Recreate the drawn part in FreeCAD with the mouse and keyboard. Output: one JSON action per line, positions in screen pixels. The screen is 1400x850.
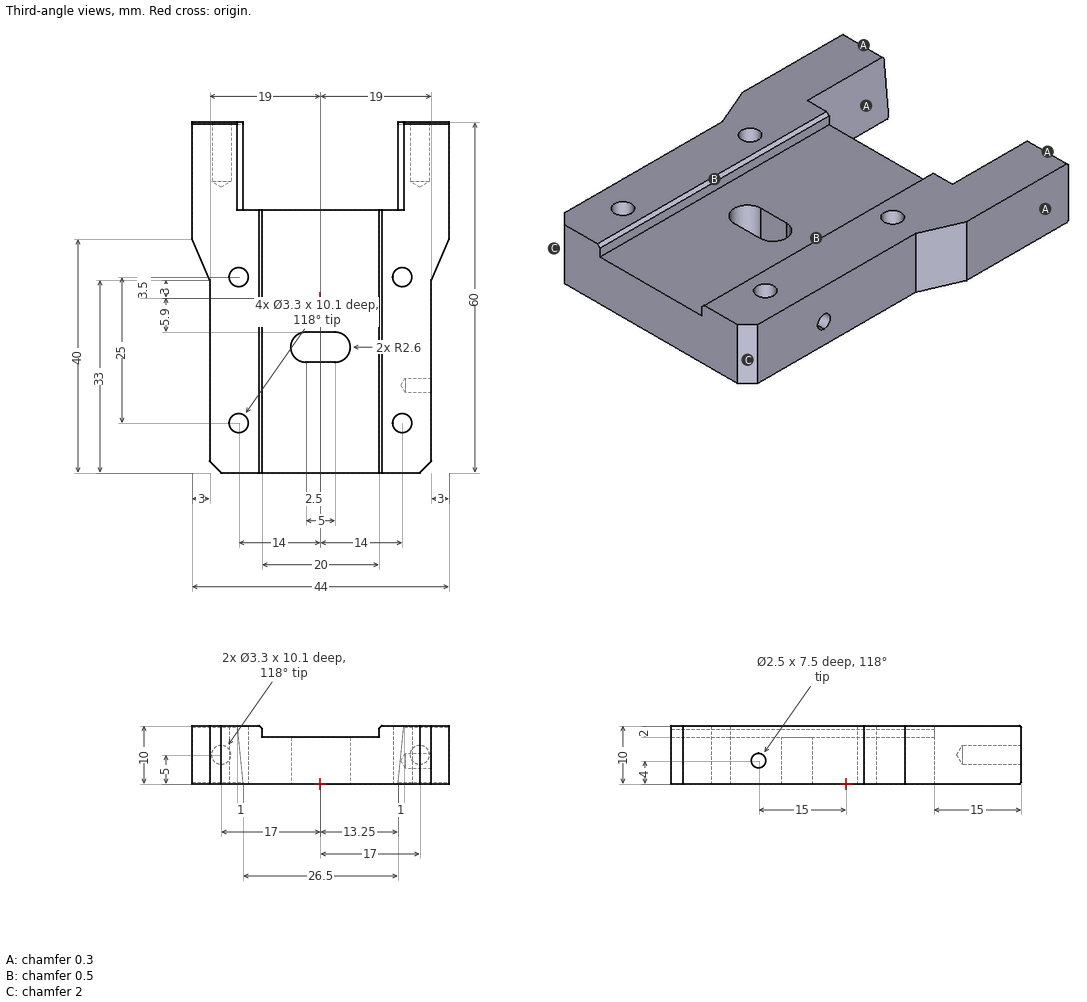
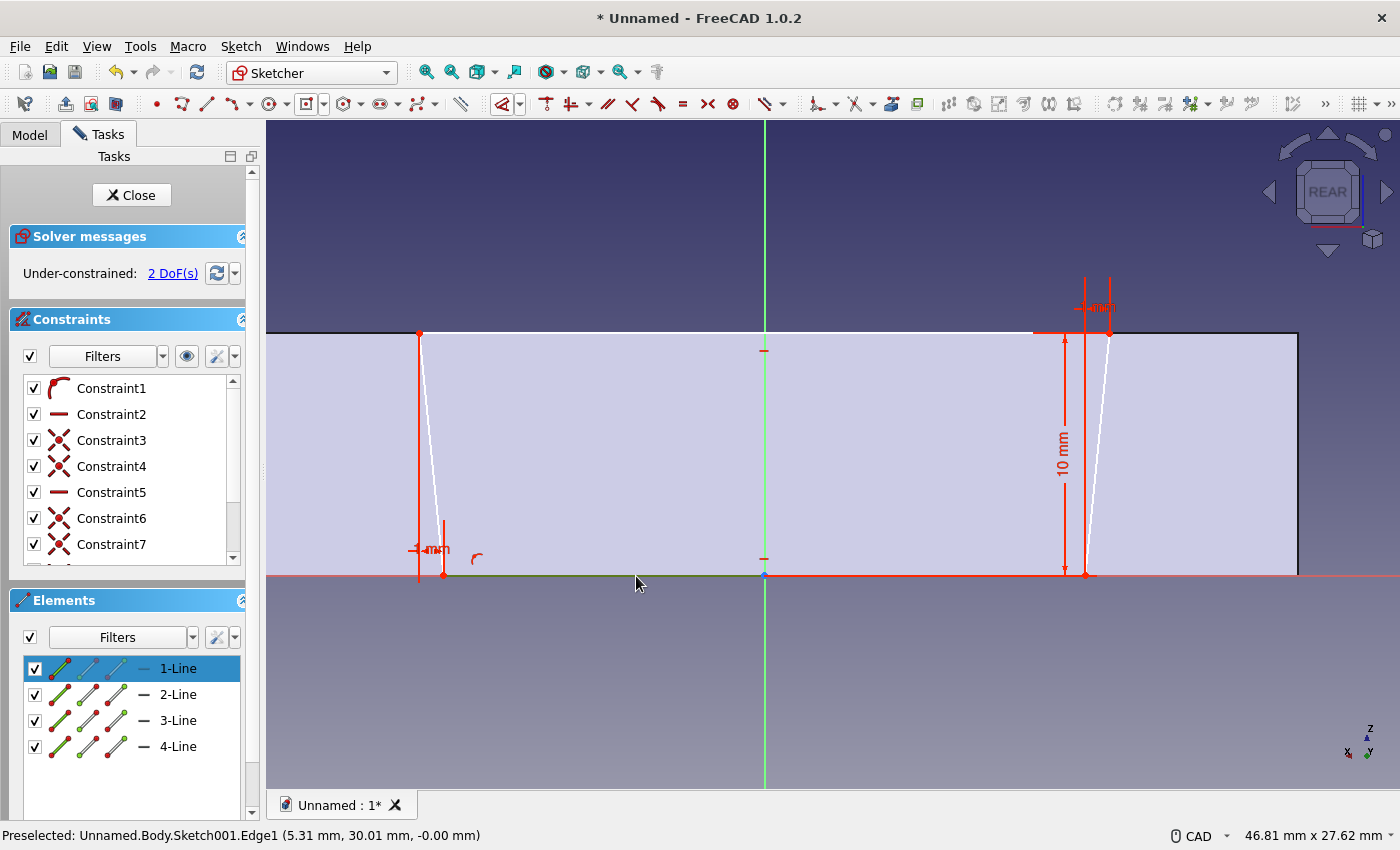
{"action": "left_click", "coordinate": [520, 104]}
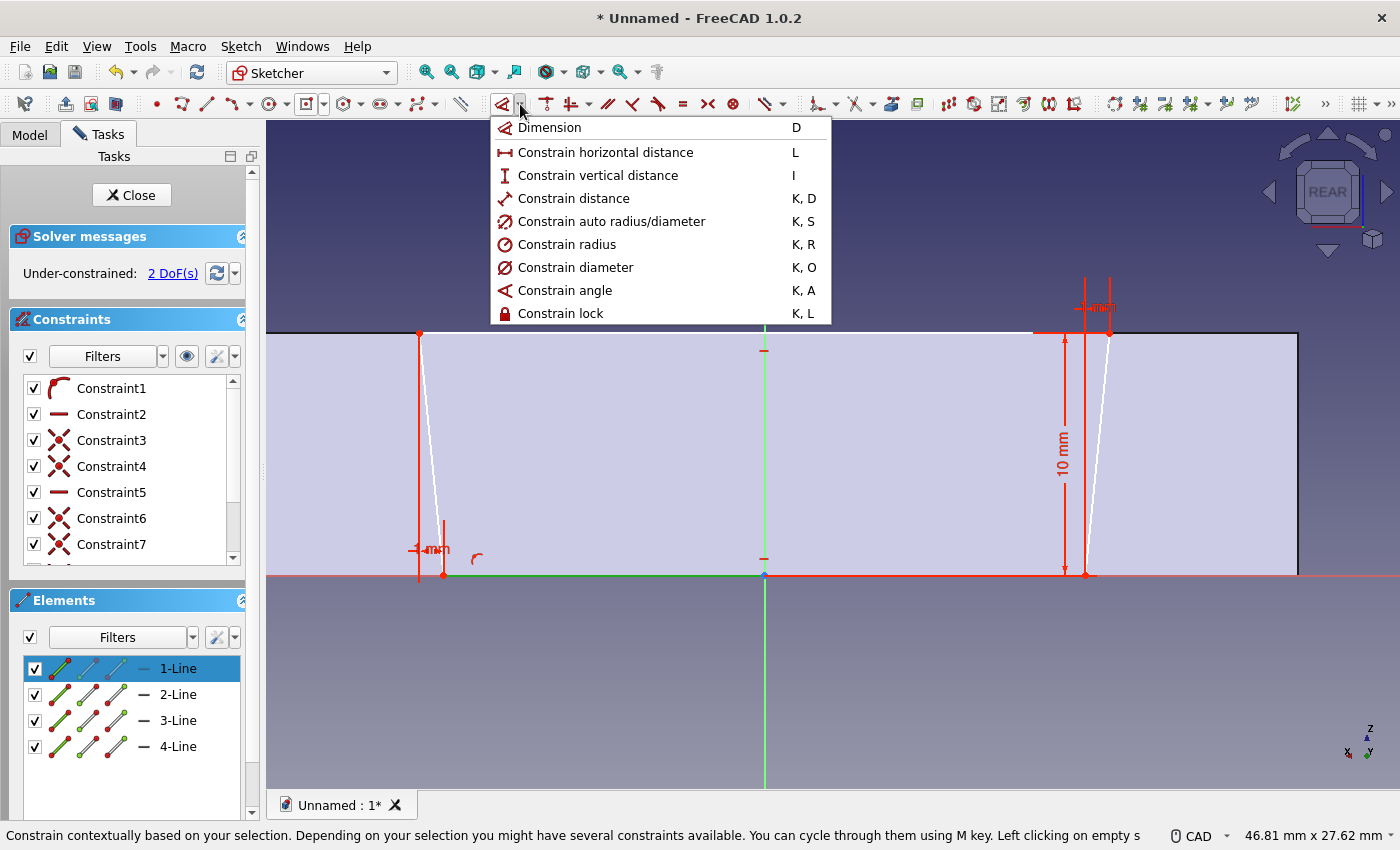
{"action": "left_click", "coordinate": [661, 152]}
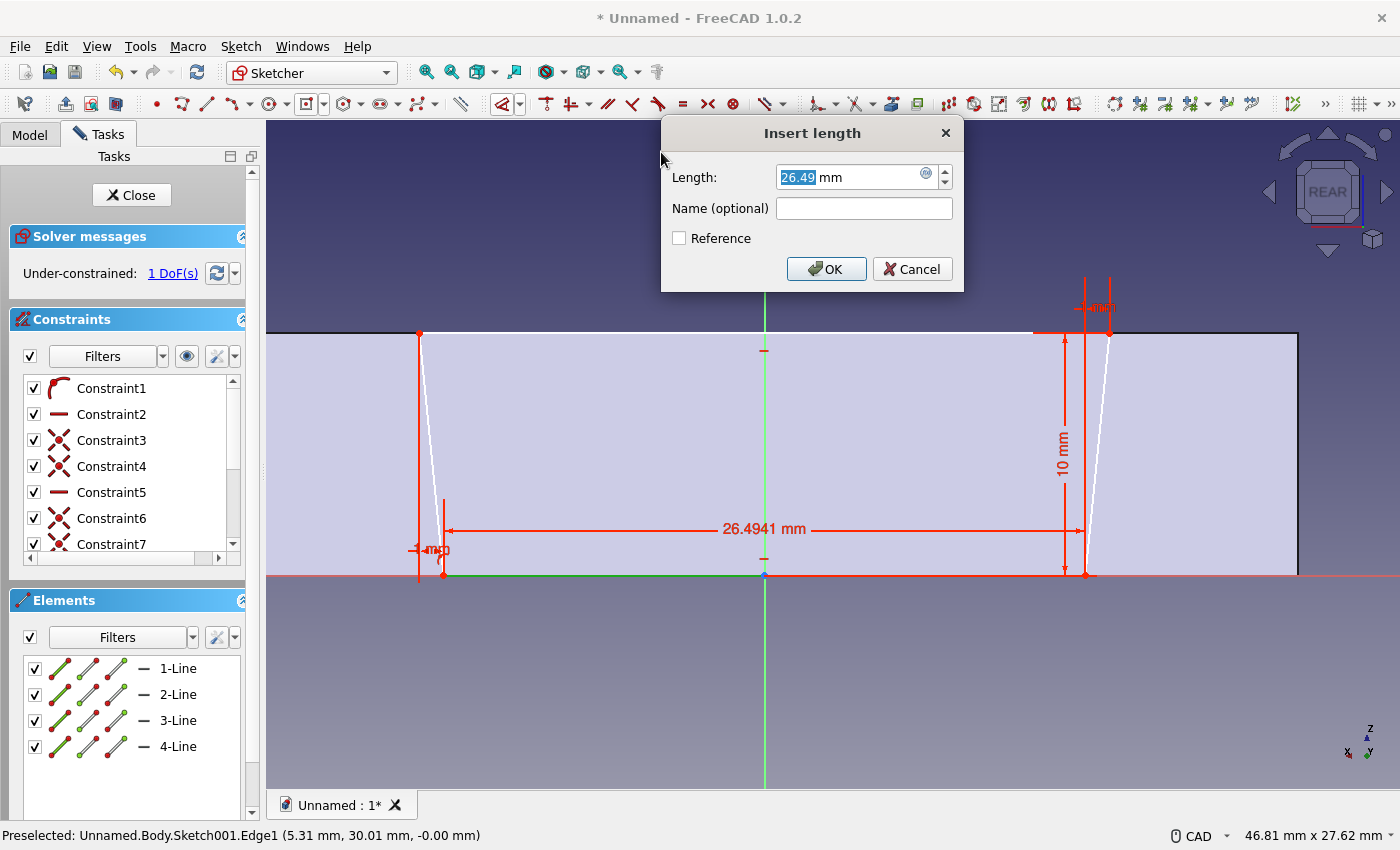
{"action": "type", "text": "26.5"}
{"action": "key", "text": "Return"}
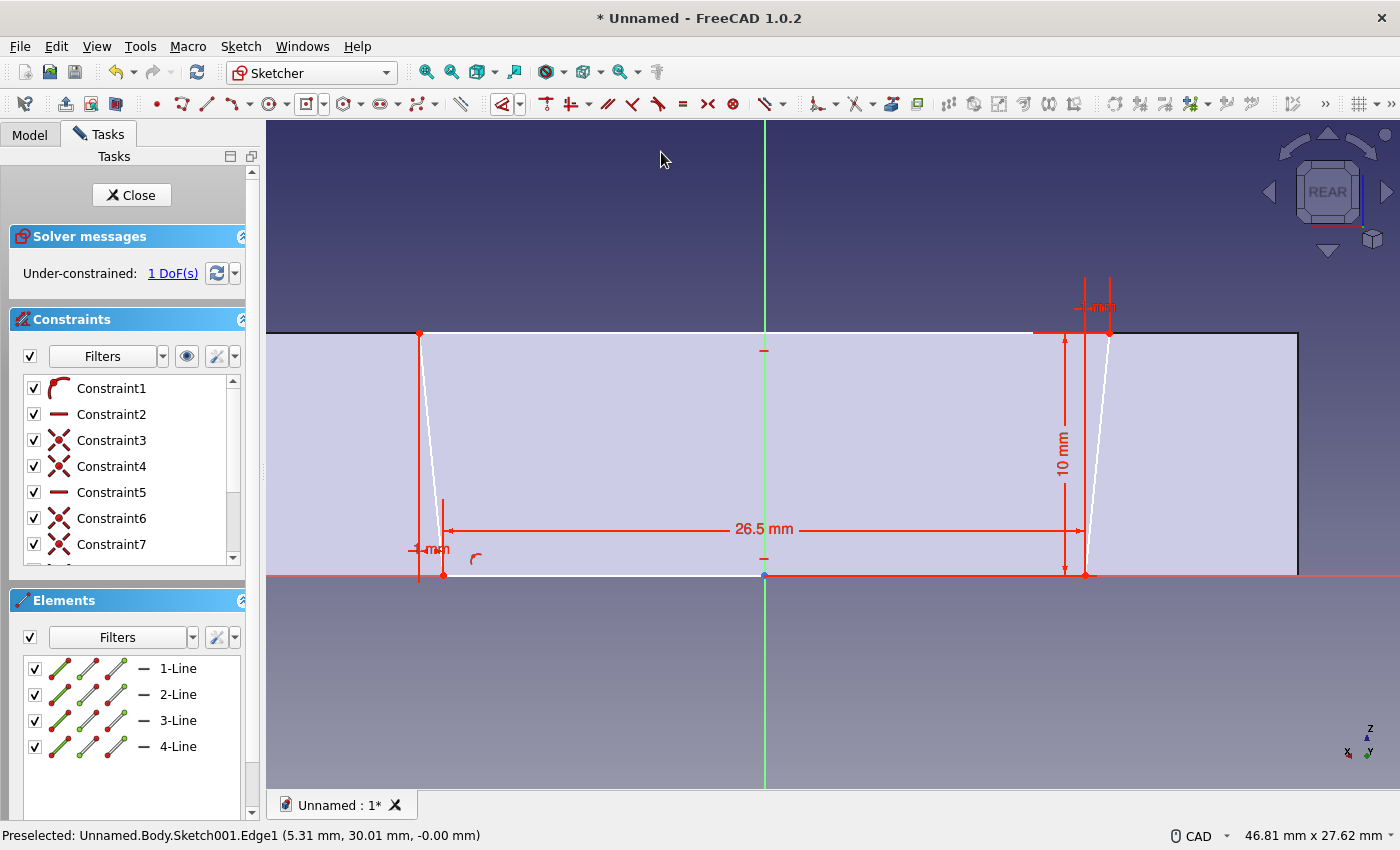
{"action": "left_click", "coordinate": [443, 576]}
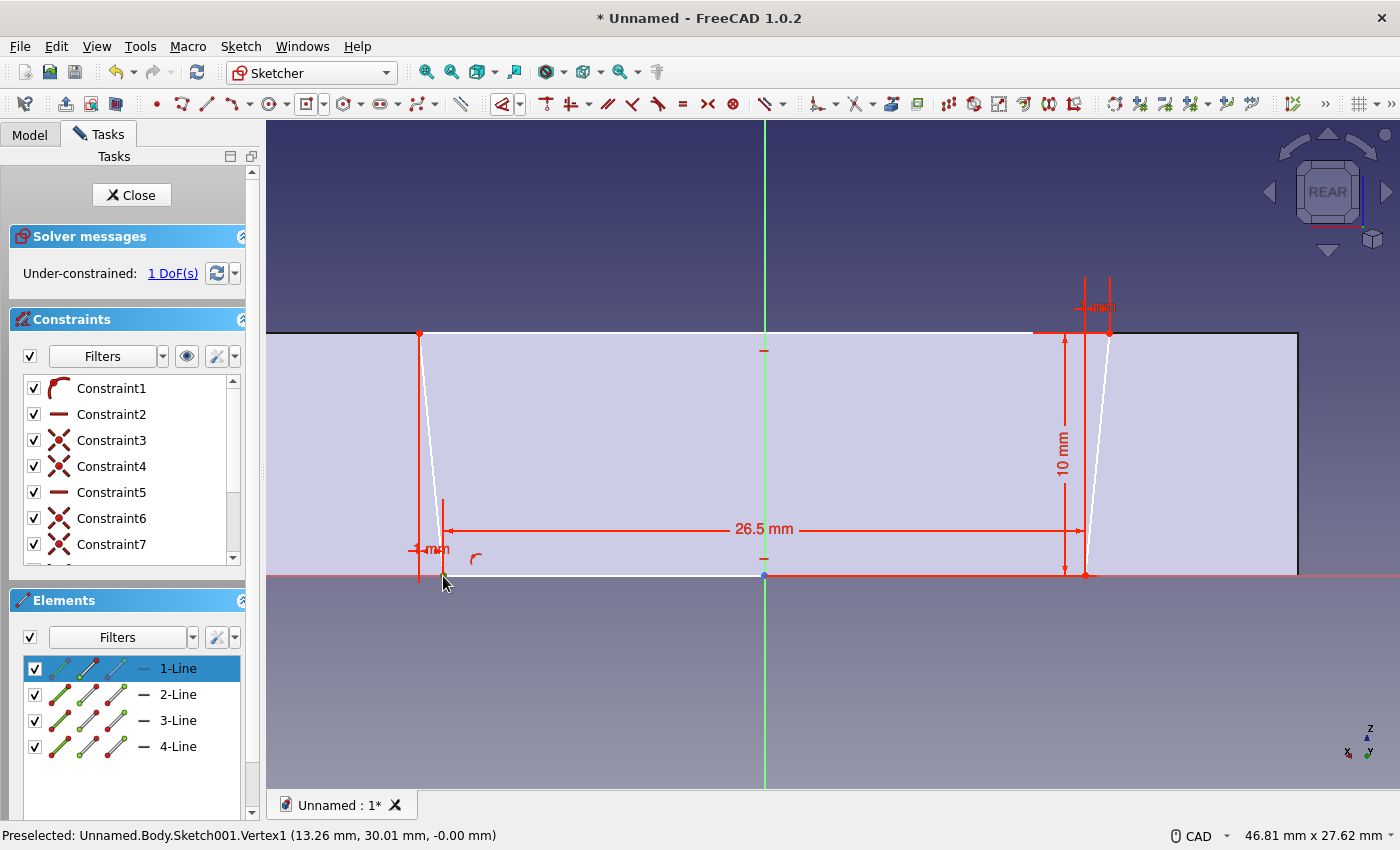
{"action": "left_click", "coordinate": [520, 104]}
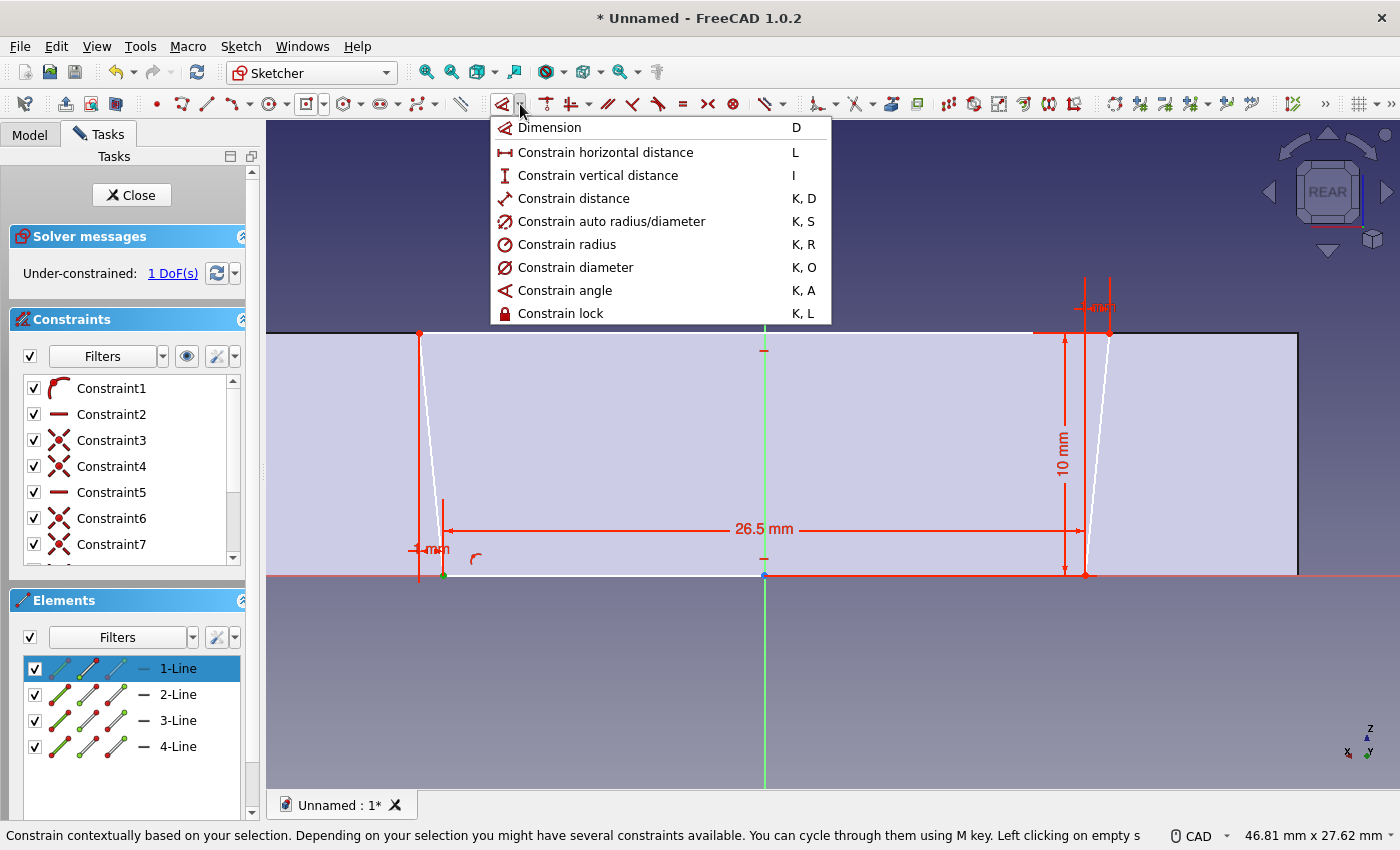
{"action": "left_click", "coordinate": [661, 152]}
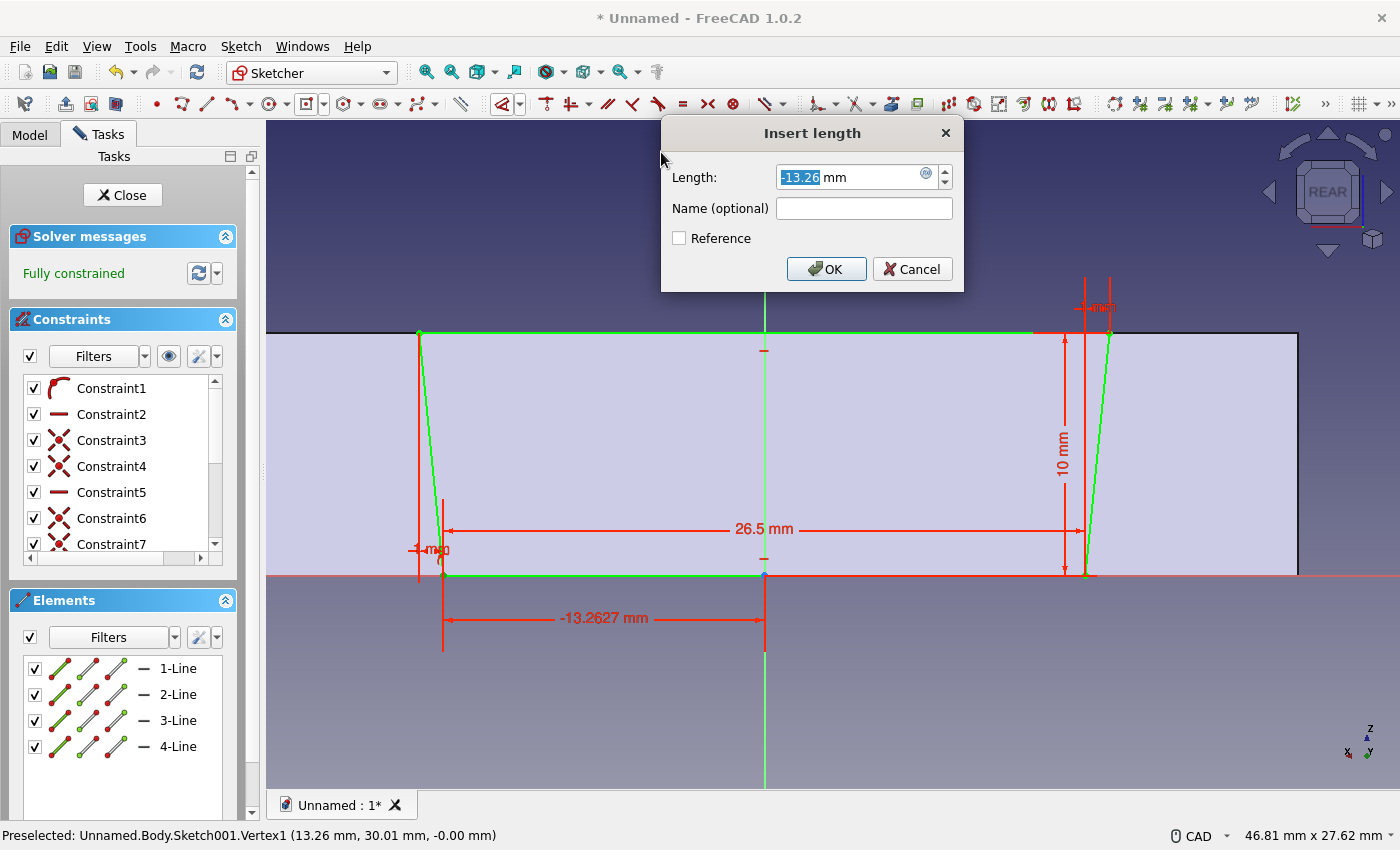
{"action": "type", "text": "-13.25"}
{"action": "key", "text": "Return"}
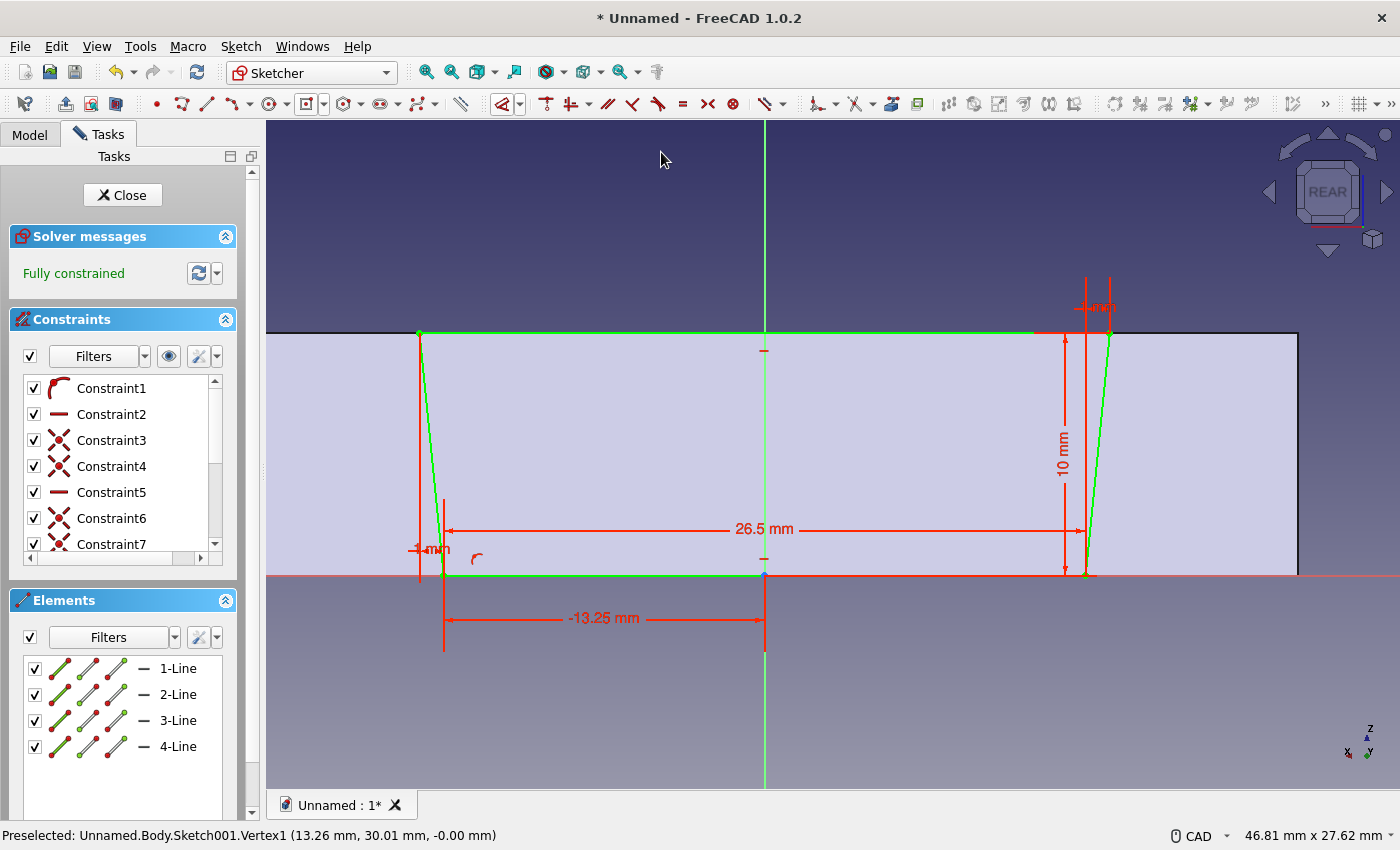
{"action": "left_click", "coordinate": [123, 195]}